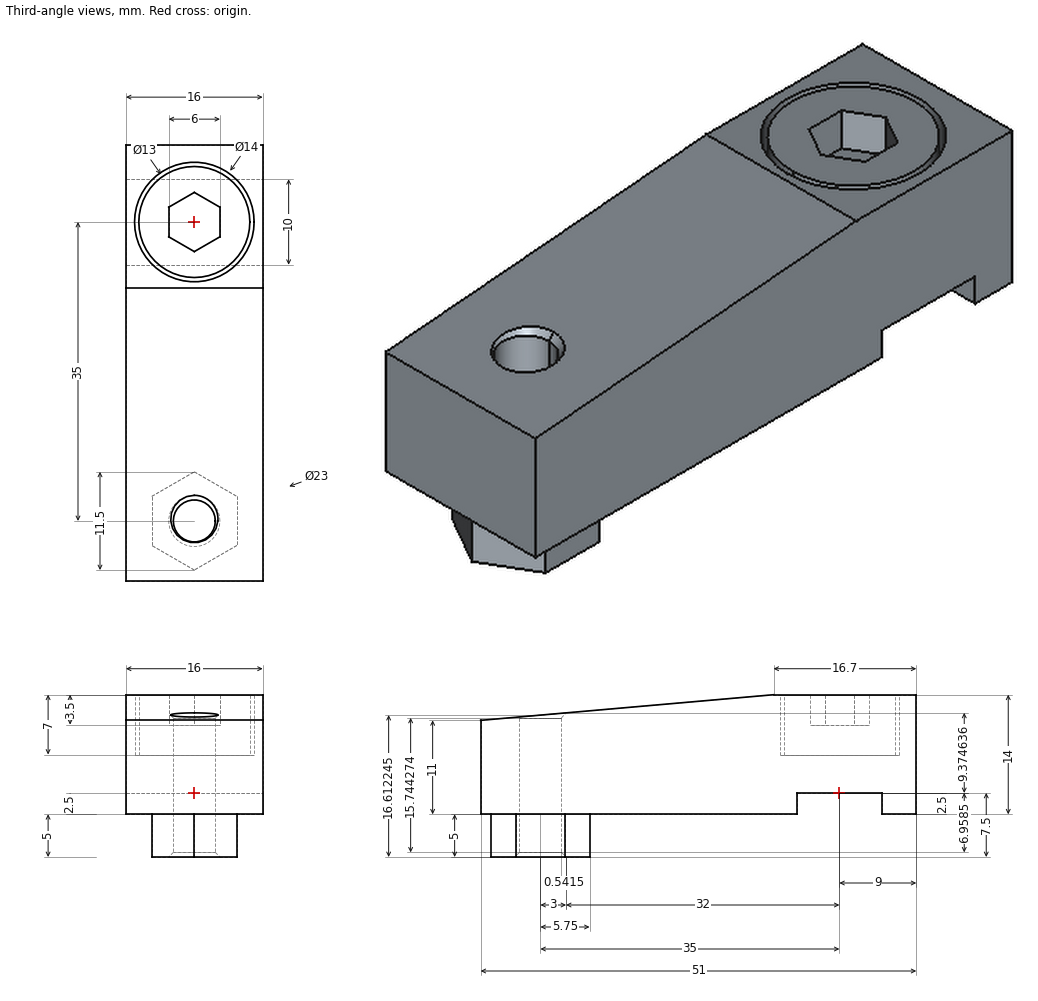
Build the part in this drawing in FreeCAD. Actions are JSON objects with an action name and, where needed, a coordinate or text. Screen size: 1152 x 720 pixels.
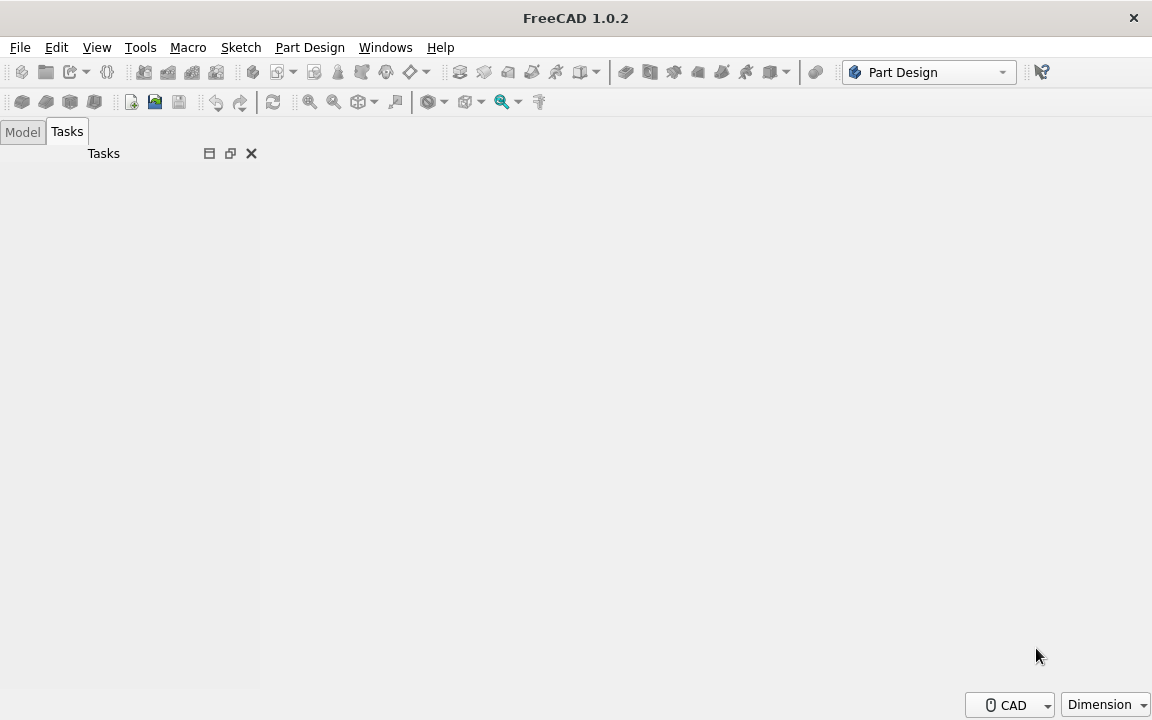
{"action": "key", "text": "ctrl+n"}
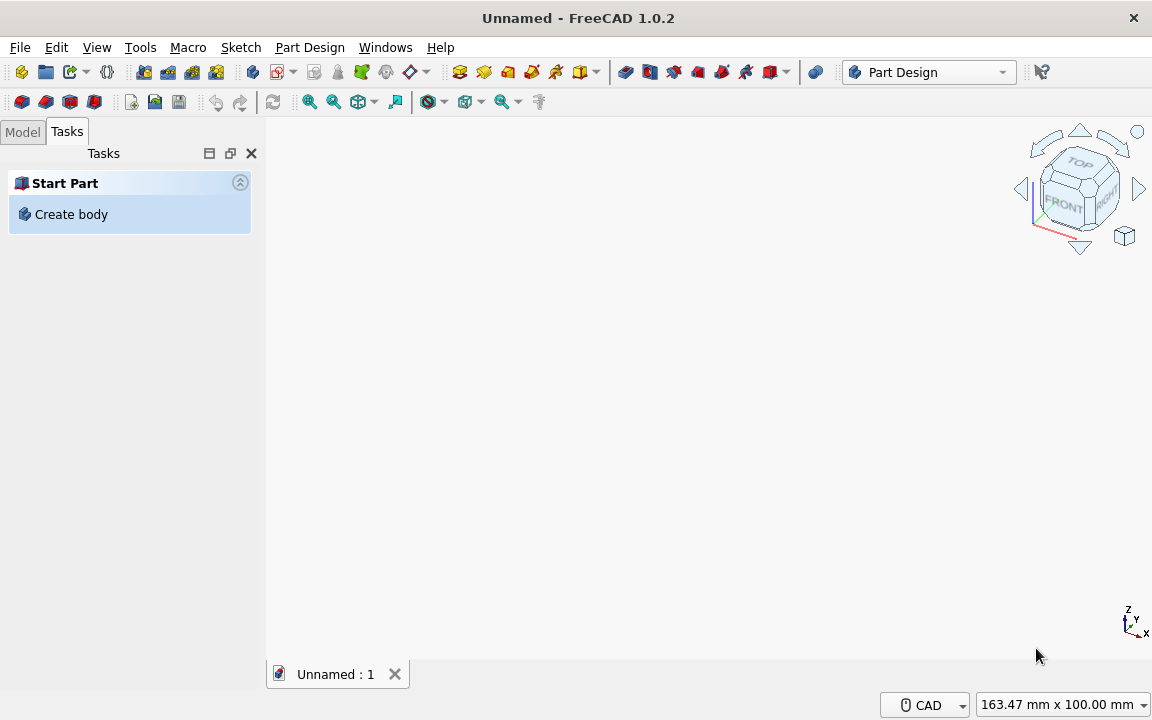
{"action": "left_click", "coordinate": [278, 72]}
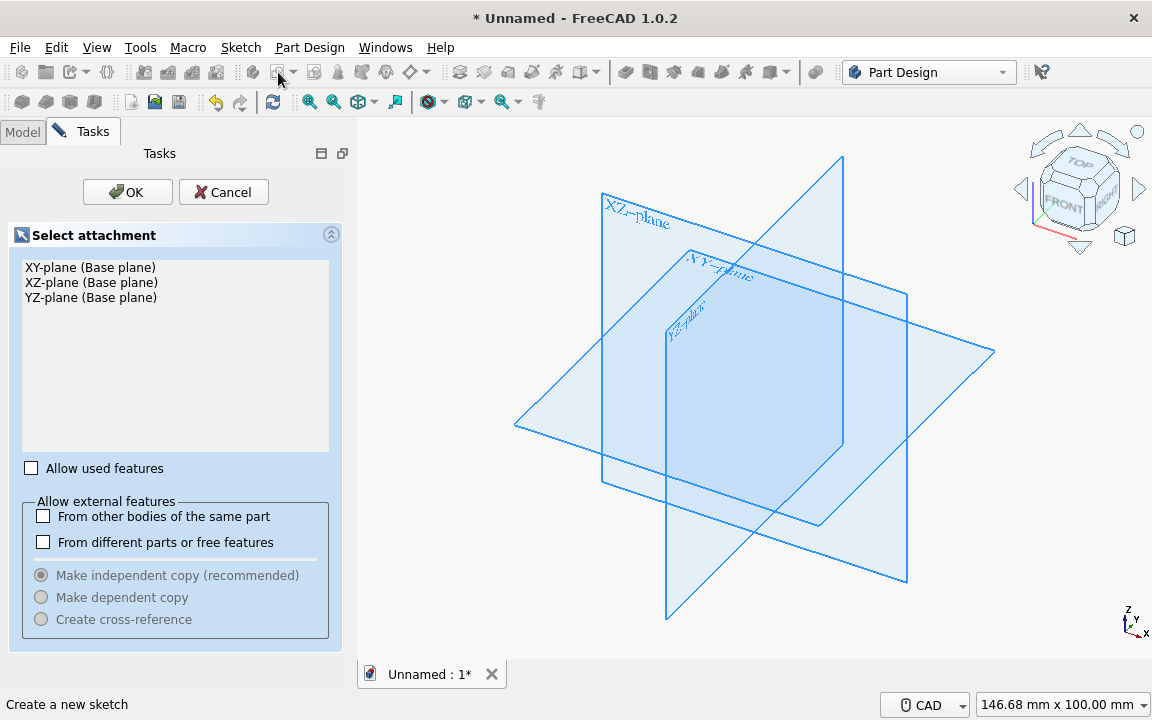
{"action": "left_click", "coordinate": [82, 298]}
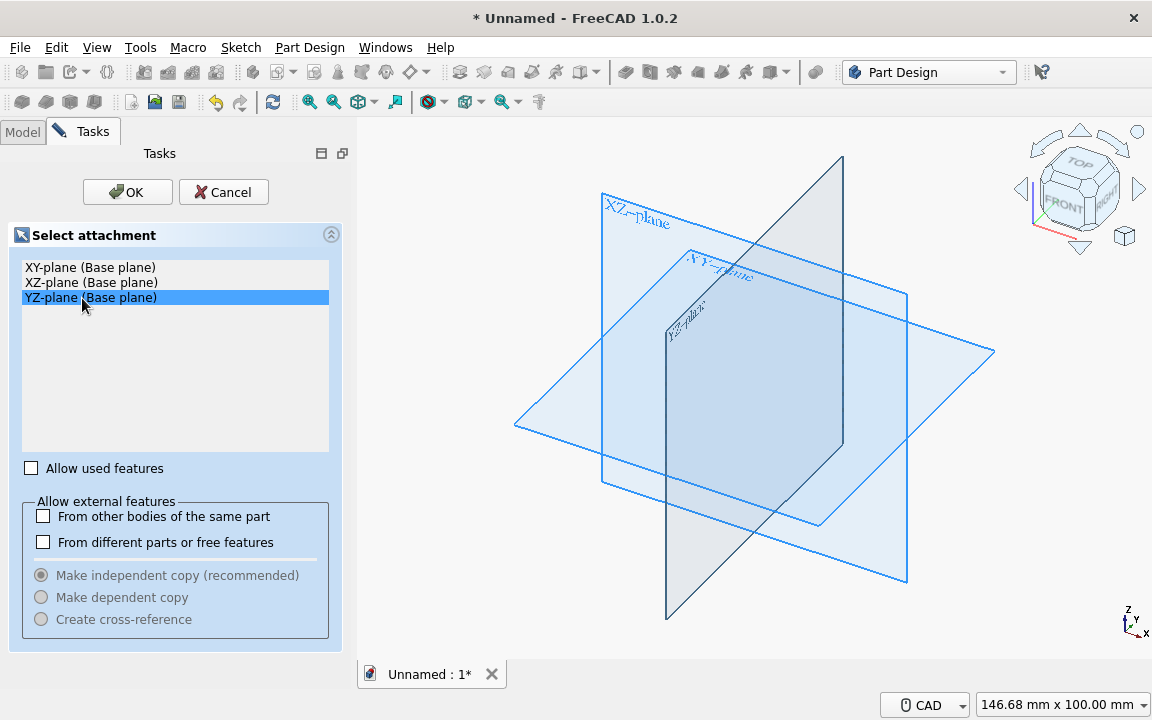
{"action": "left_click", "coordinate": [128, 192]}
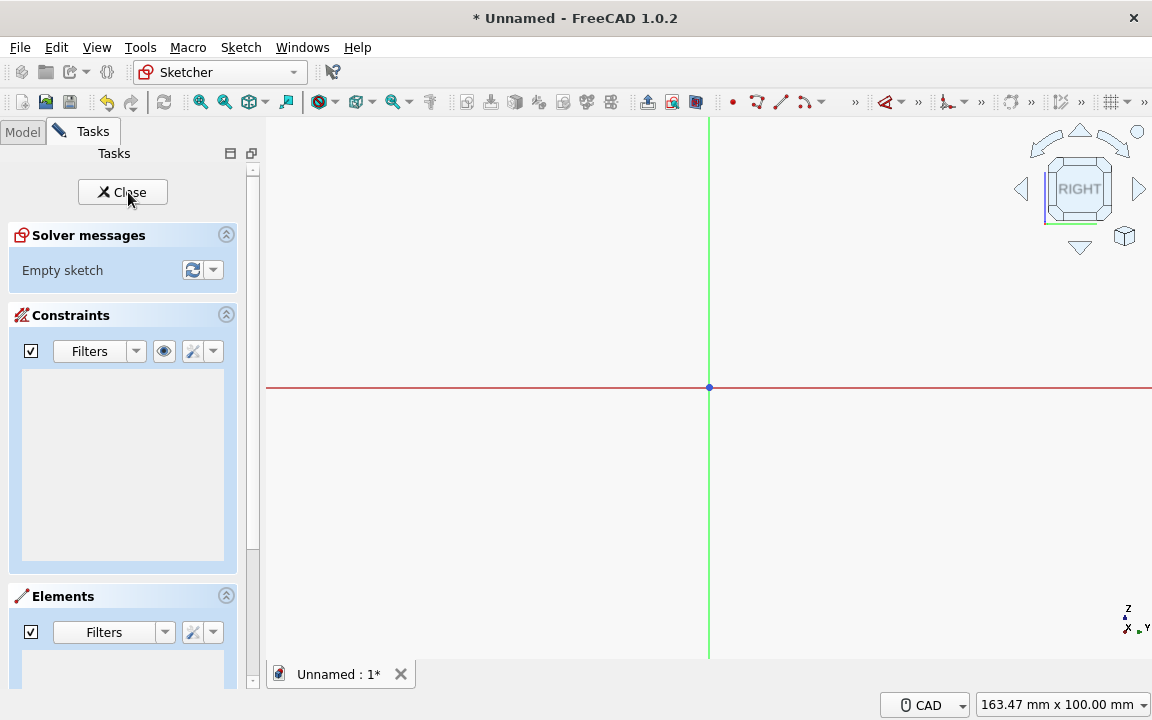
{"action": "scroll", "coordinate": [594, 334], "scroll_direction": "up", "scroll_amount": 3}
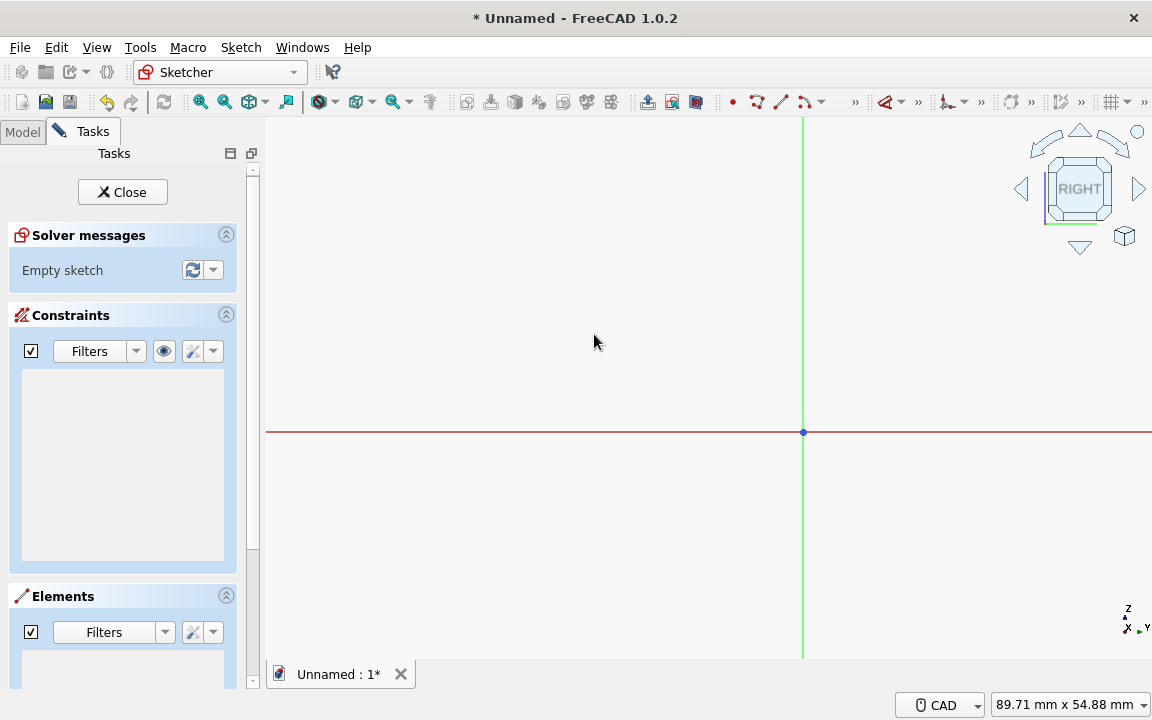
{"action": "left_click", "coordinate": [758, 102]}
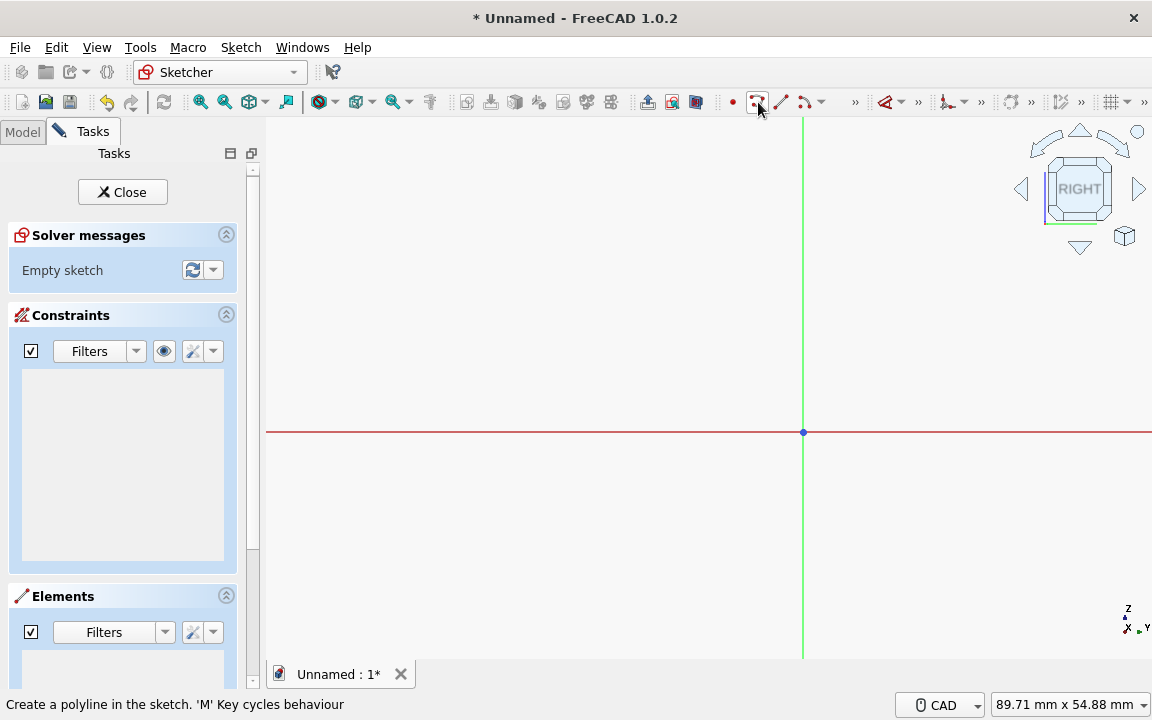
{"action": "left_click", "coordinate": [892, 457]}
{"action": "left_click", "coordinate": [892, 318]}
{"action": "left_click", "coordinate": [727, 318]}
{"action": "left_click", "coordinate": [388, 348]}
{"action": "left_click", "coordinate": [388, 457]}
{"action": "left_click", "coordinate": [892, 458]}
{"action": "key", "text": "Escape"}
{"action": "key", "text": "Escape"}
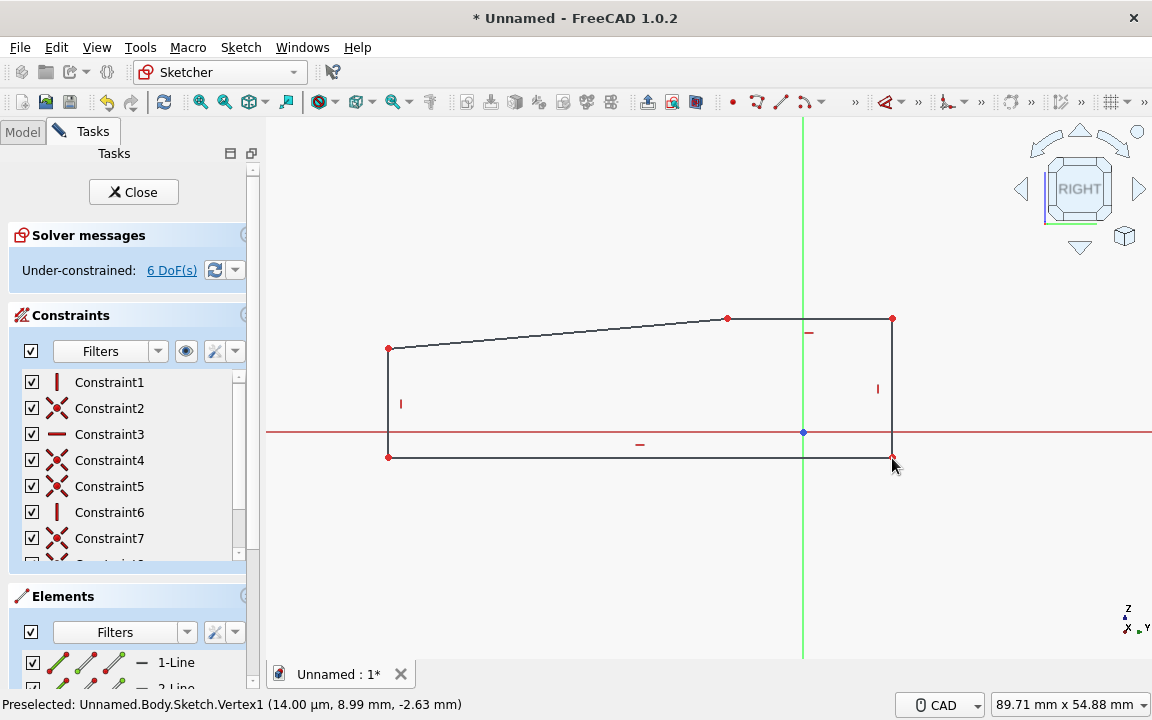
{"action": "left_click", "coordinate": [892, 416]}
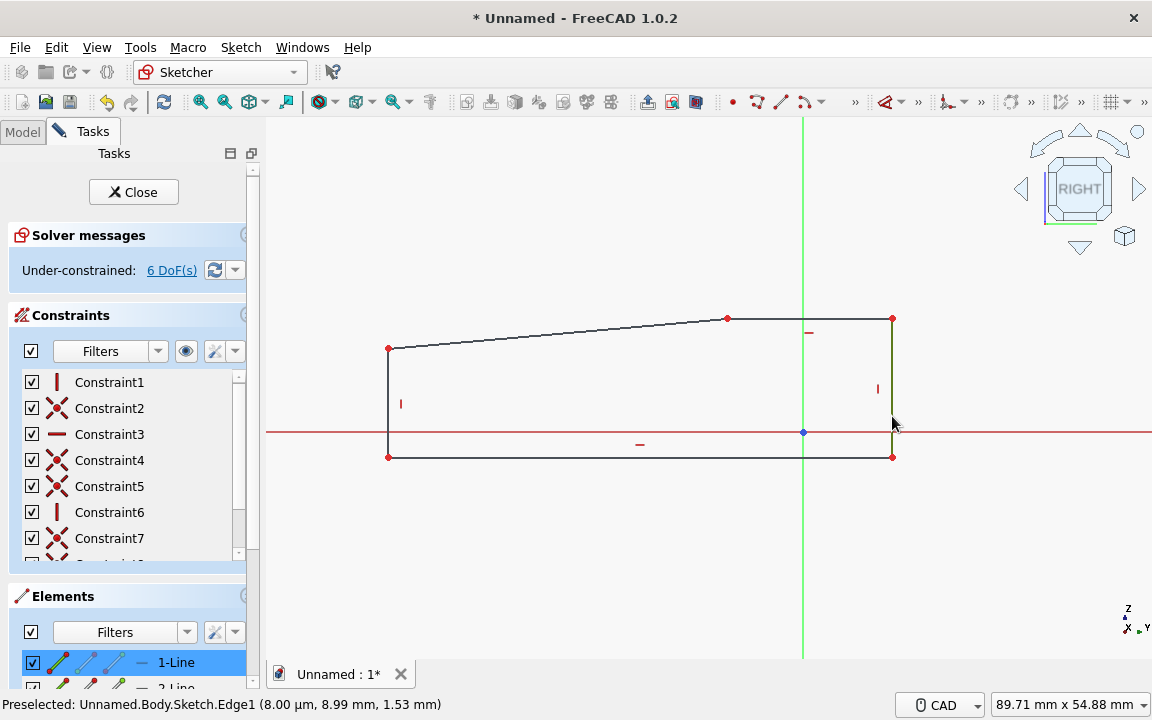
{"action": "key", "text": "i"}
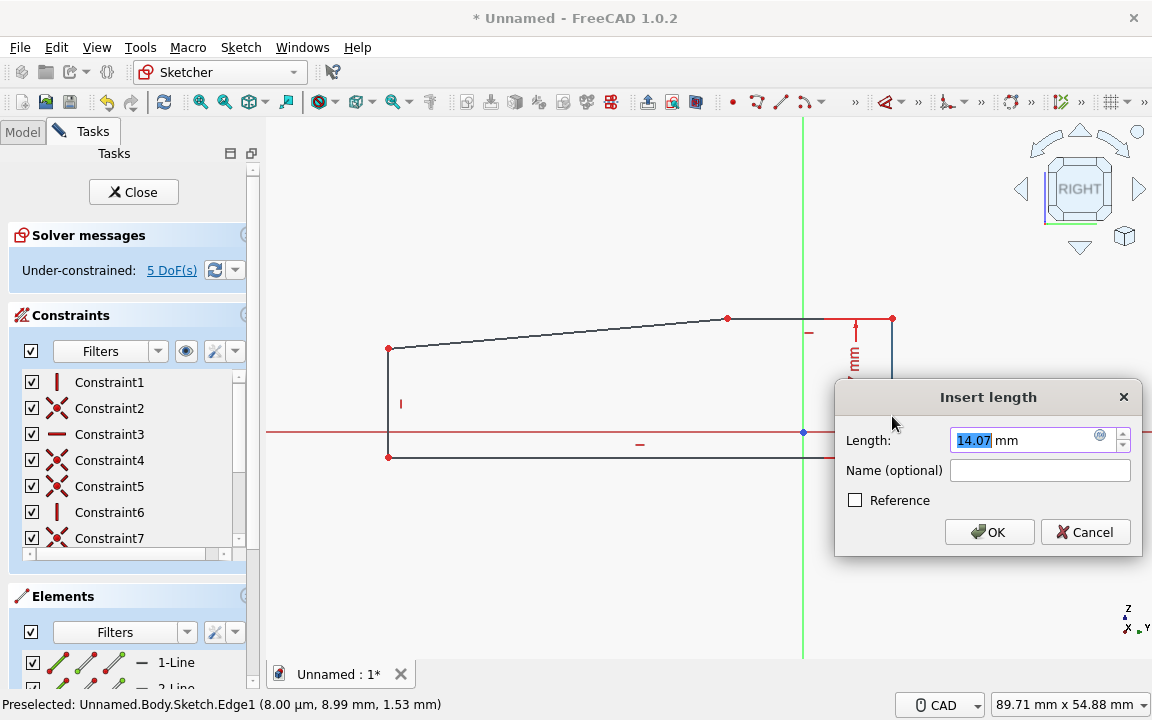
{"action": "type", "text": "14"}
{"action": "key", "text": "Return"}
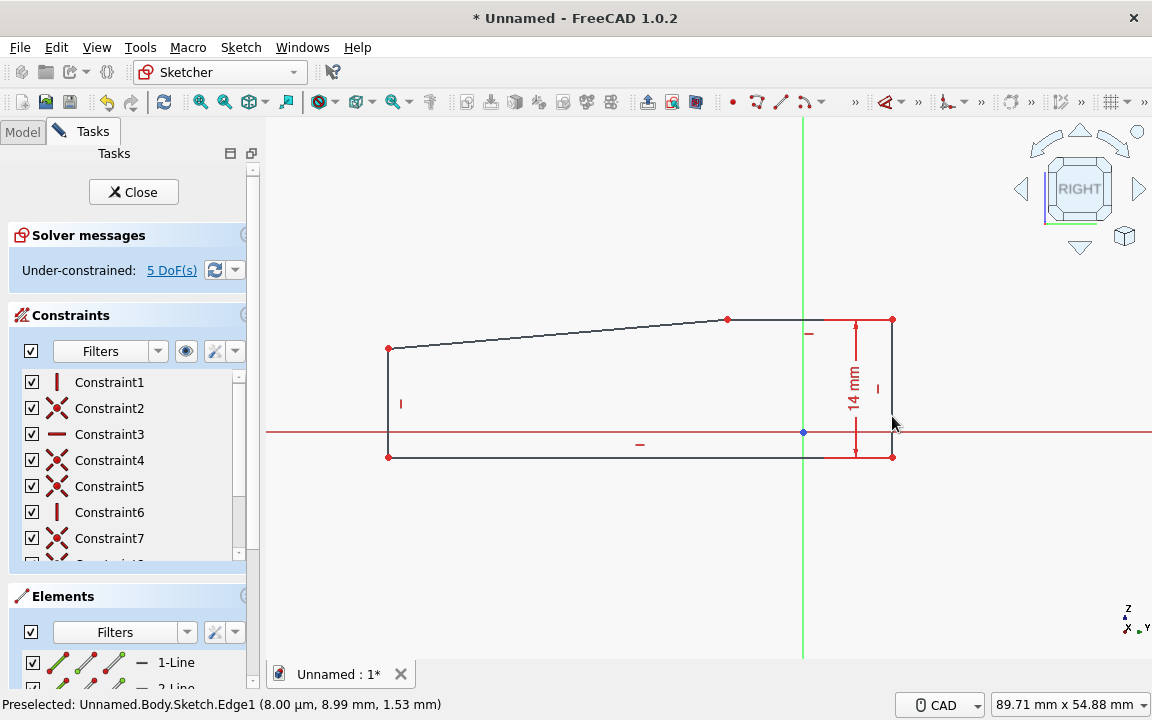
{"action": "left_click", "coordinate": [388, 382]}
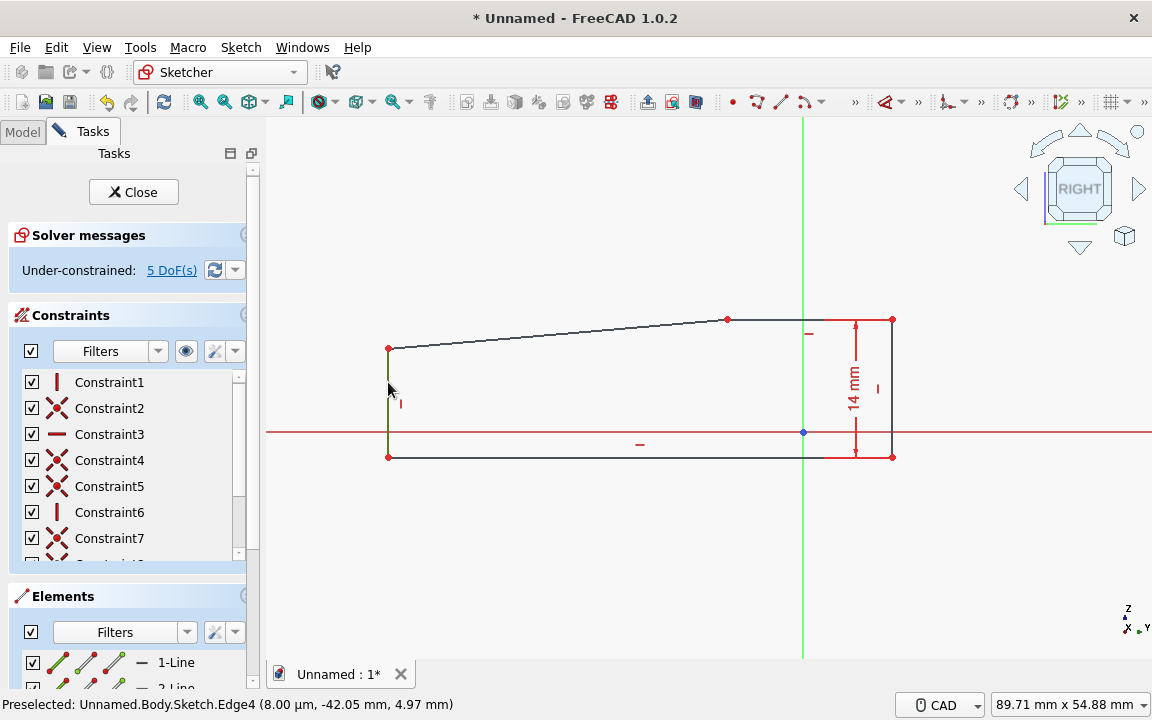
{"action": "key", "text": "i"}